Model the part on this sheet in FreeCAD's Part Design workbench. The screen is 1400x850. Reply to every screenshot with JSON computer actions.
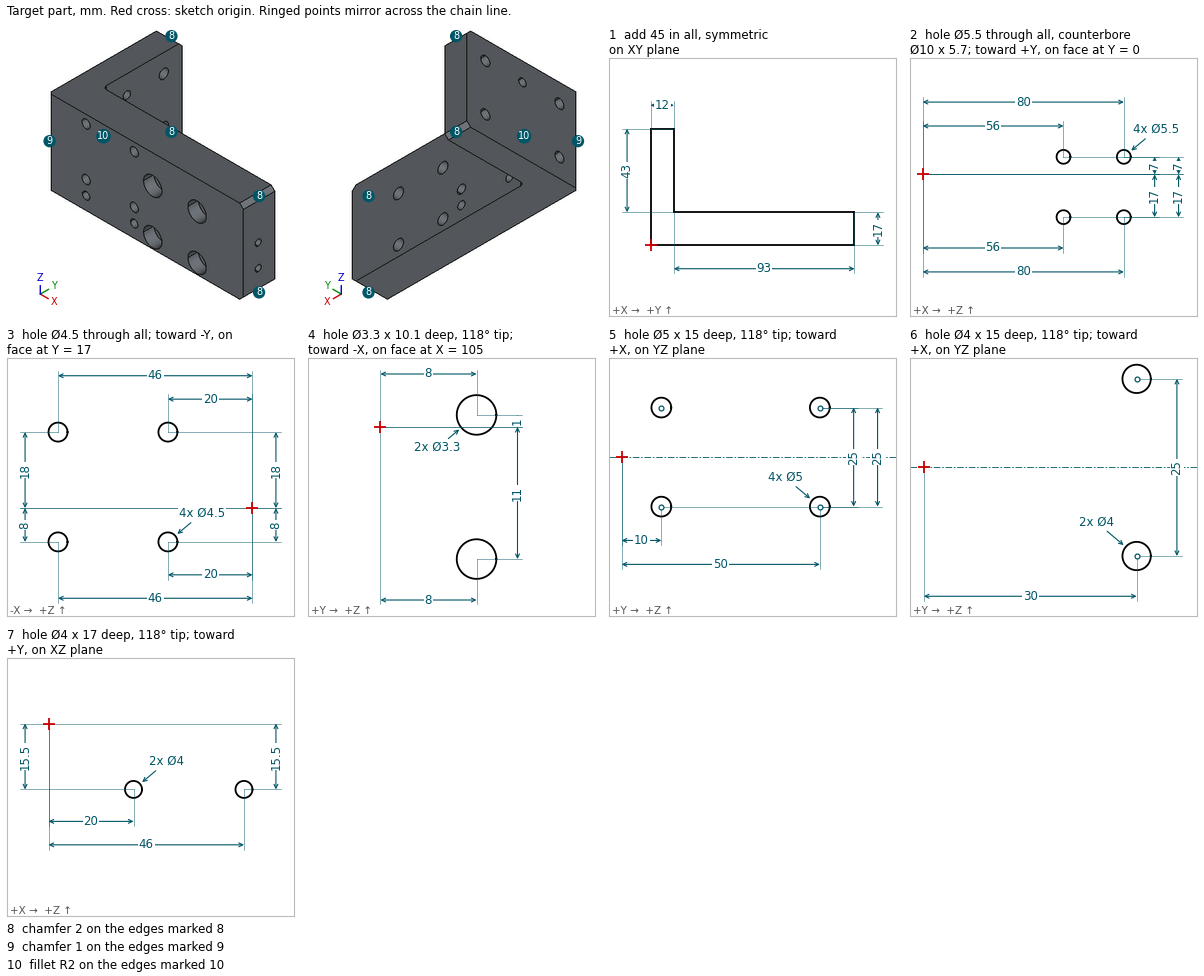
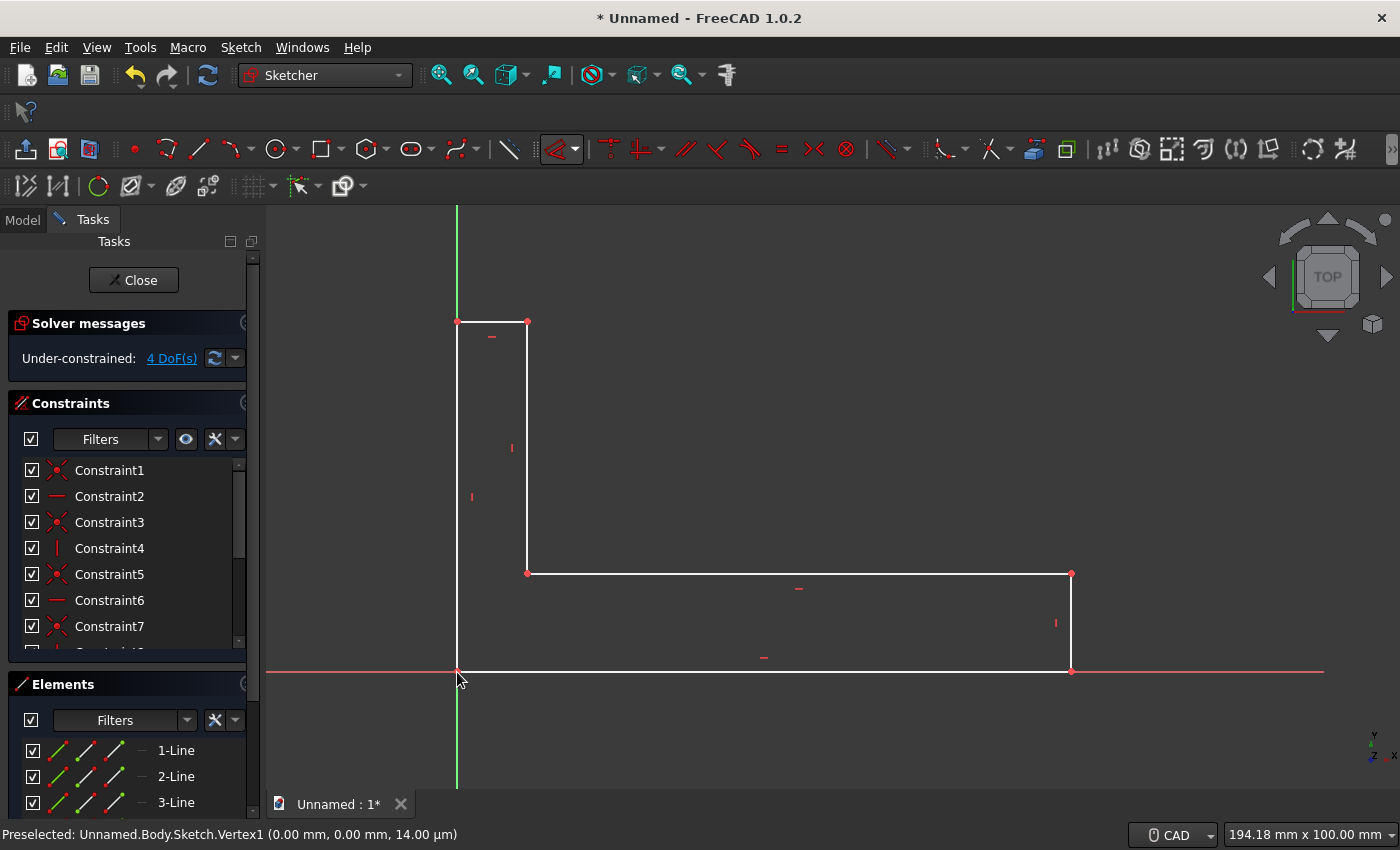
{"action": "left_click", "coordinate": [1071, 643]}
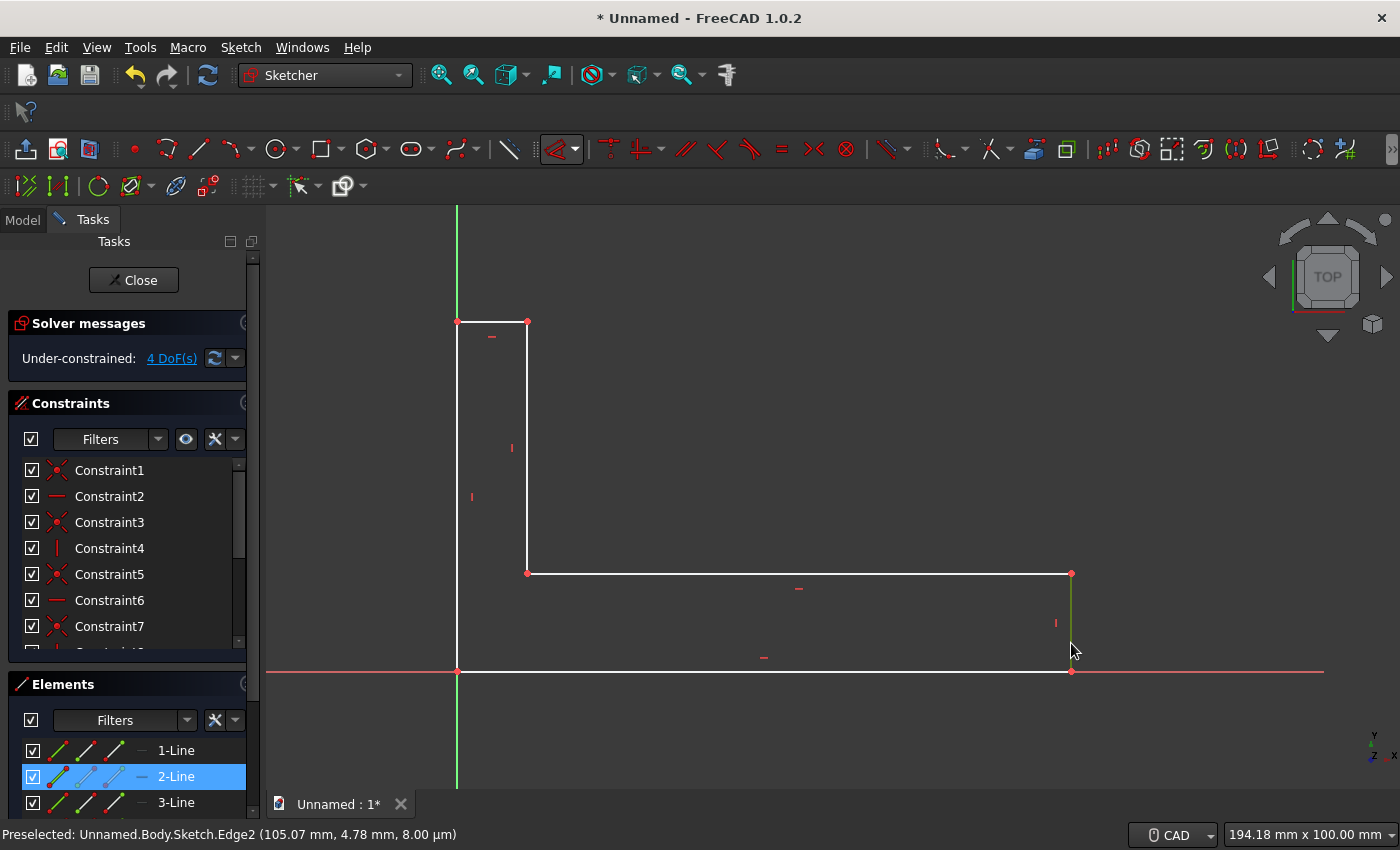
{"action": "key", "text": "i"}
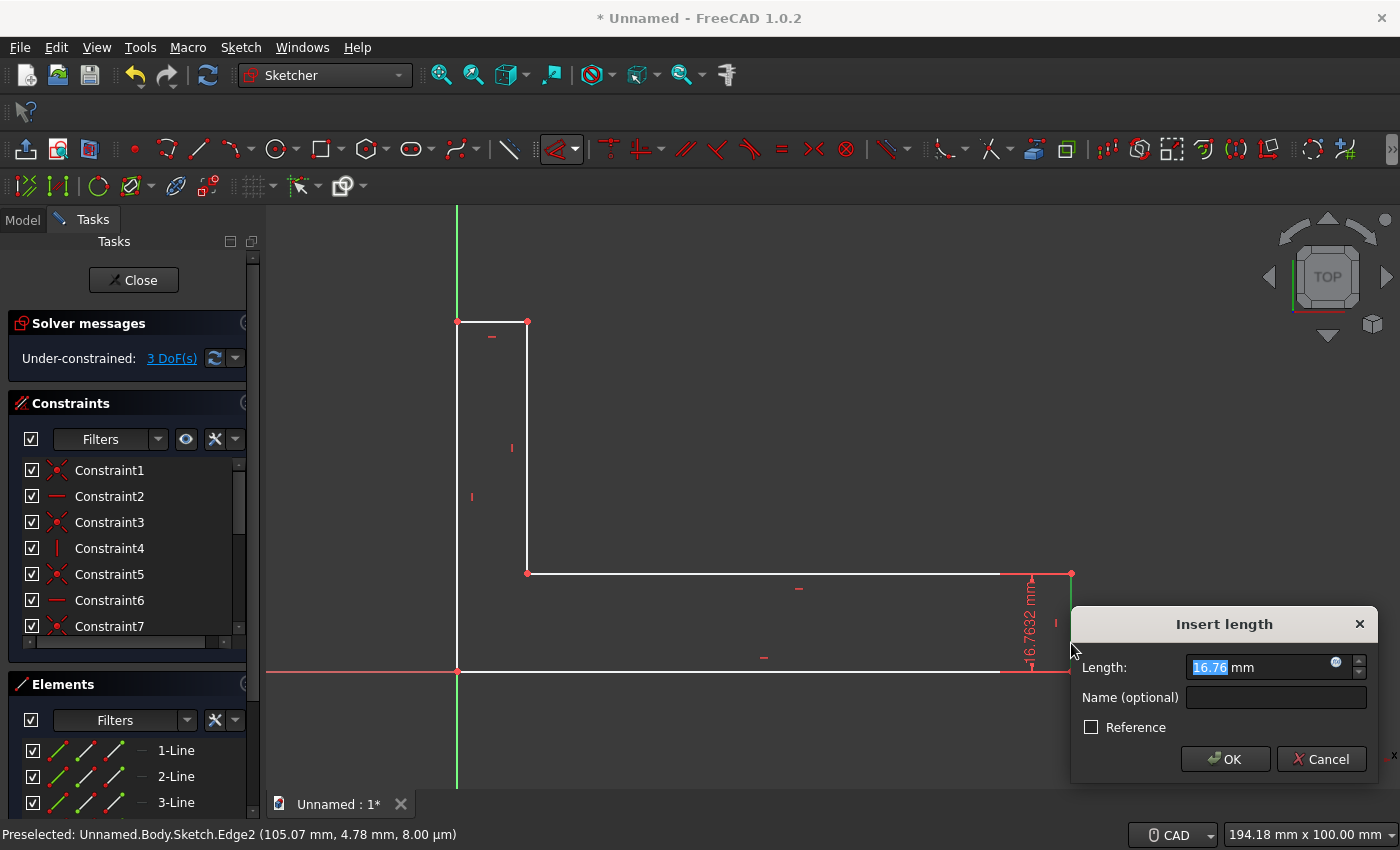
{"action": "type", "text": "17"}
{"action": "key", "text": "Return"}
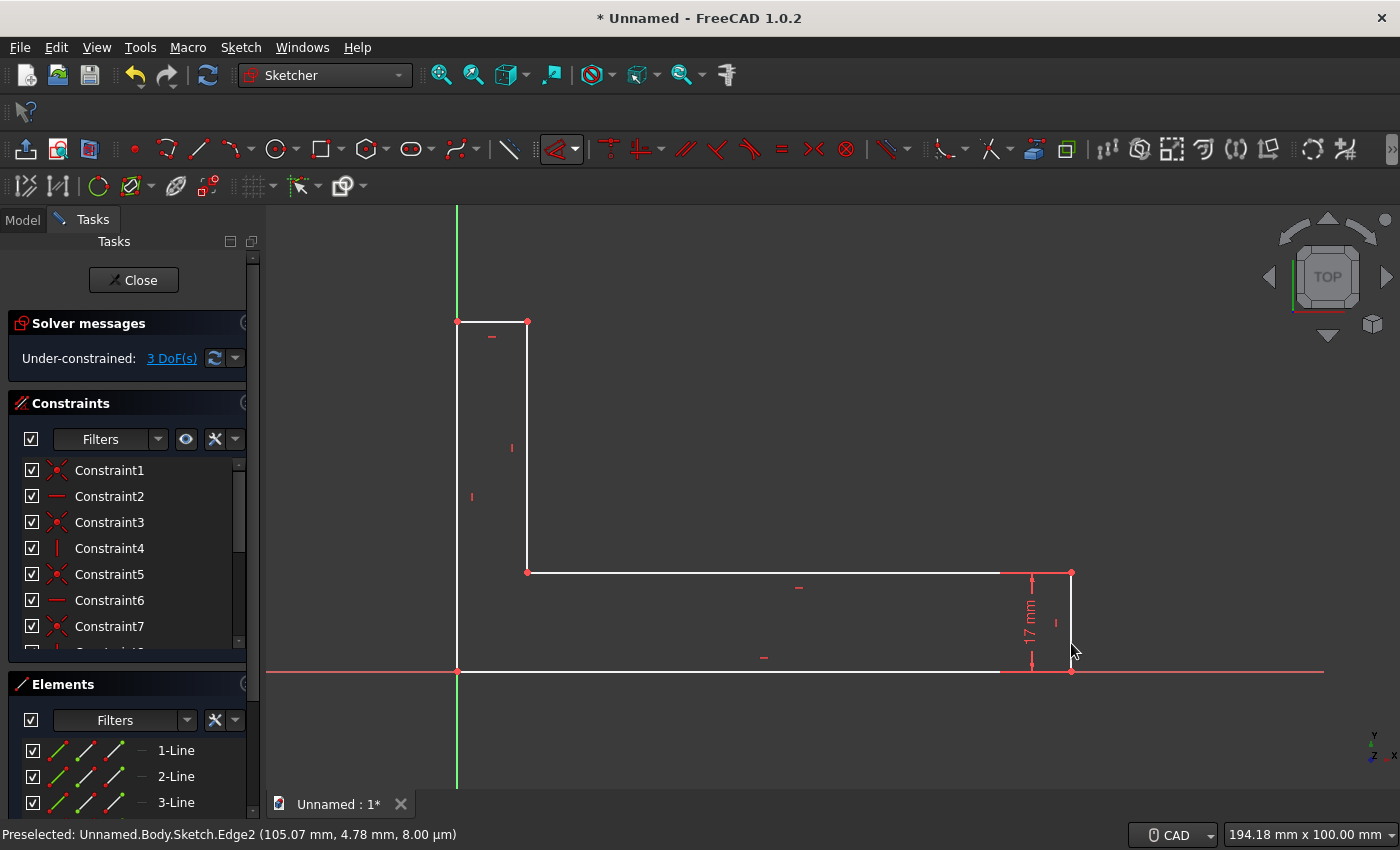
{"action": "left_click", "coordinate": [908, 573]}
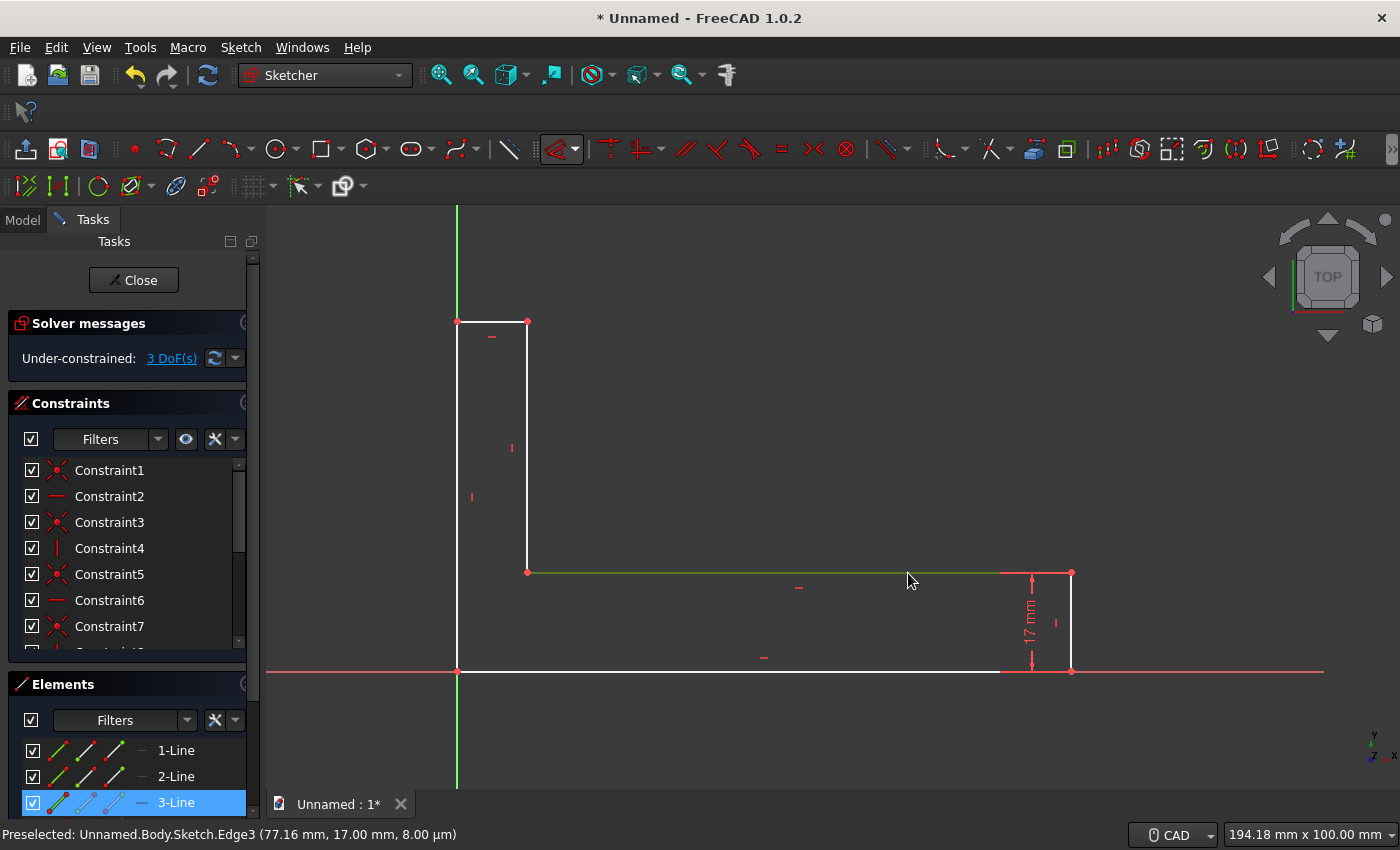
{"action": "key", "text": "l"}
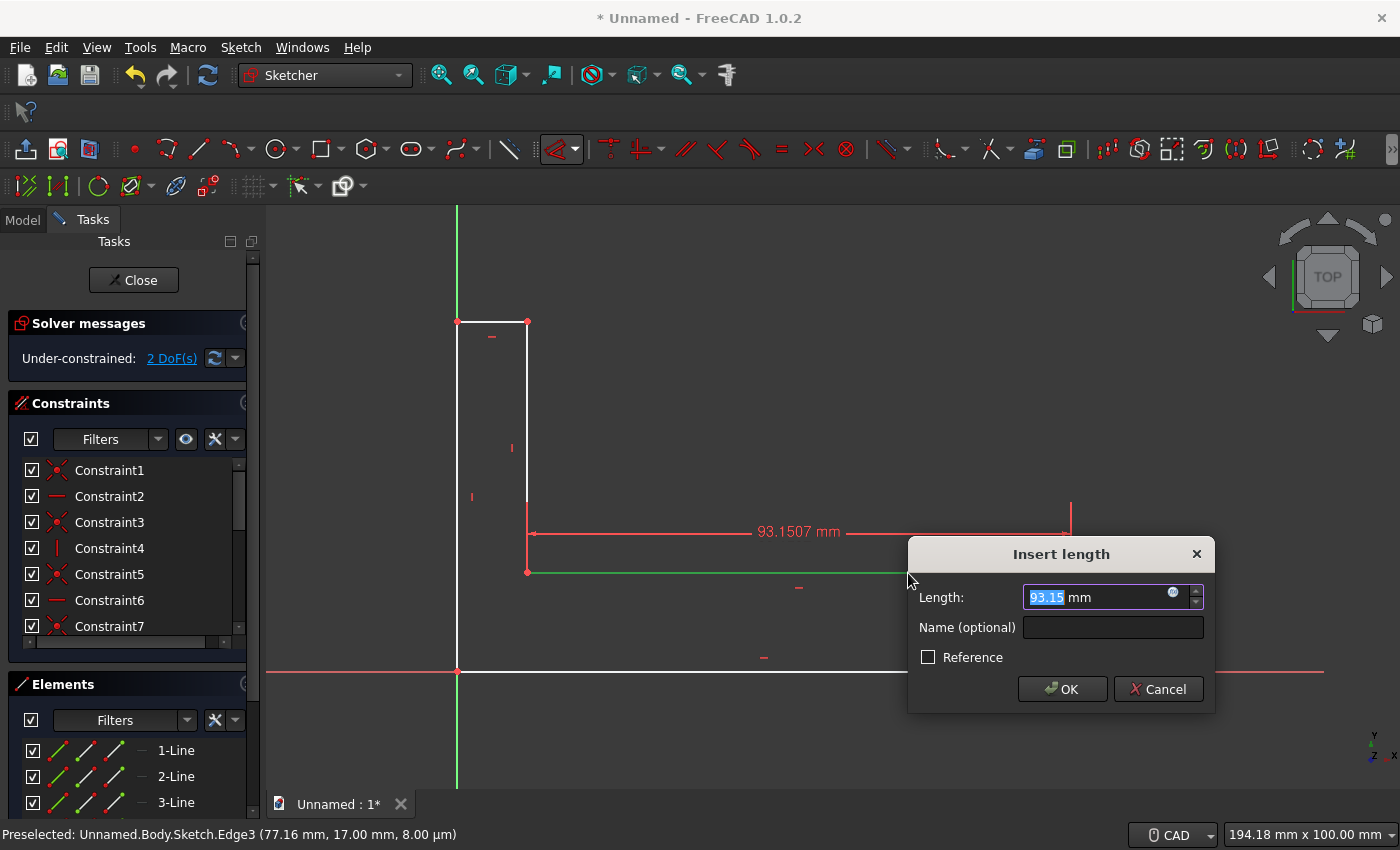
{"action": "type", "text": "93"}
{"action": "key", "text": "Return"}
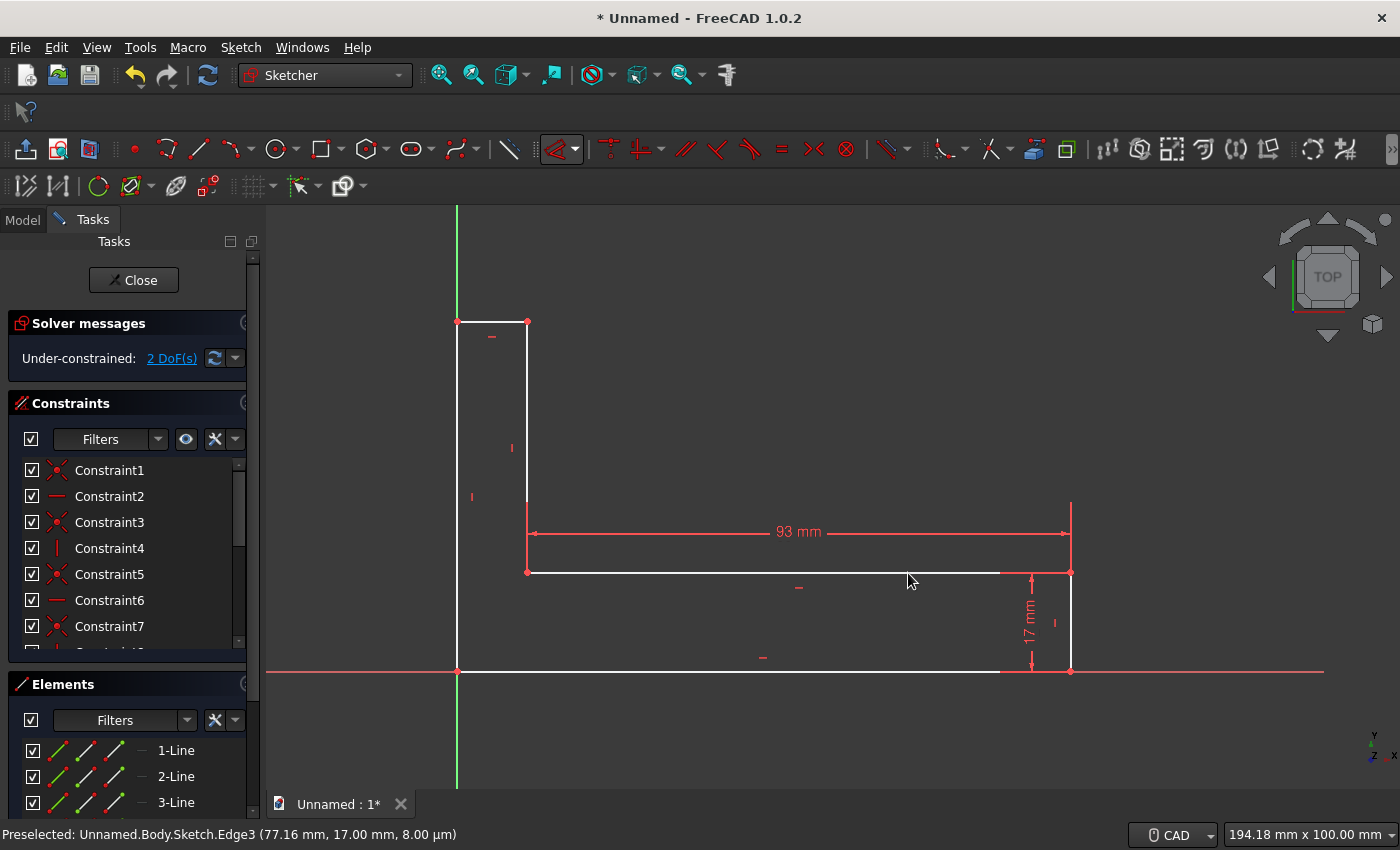
{"action": "left_click", "coordinate": [527, 497]}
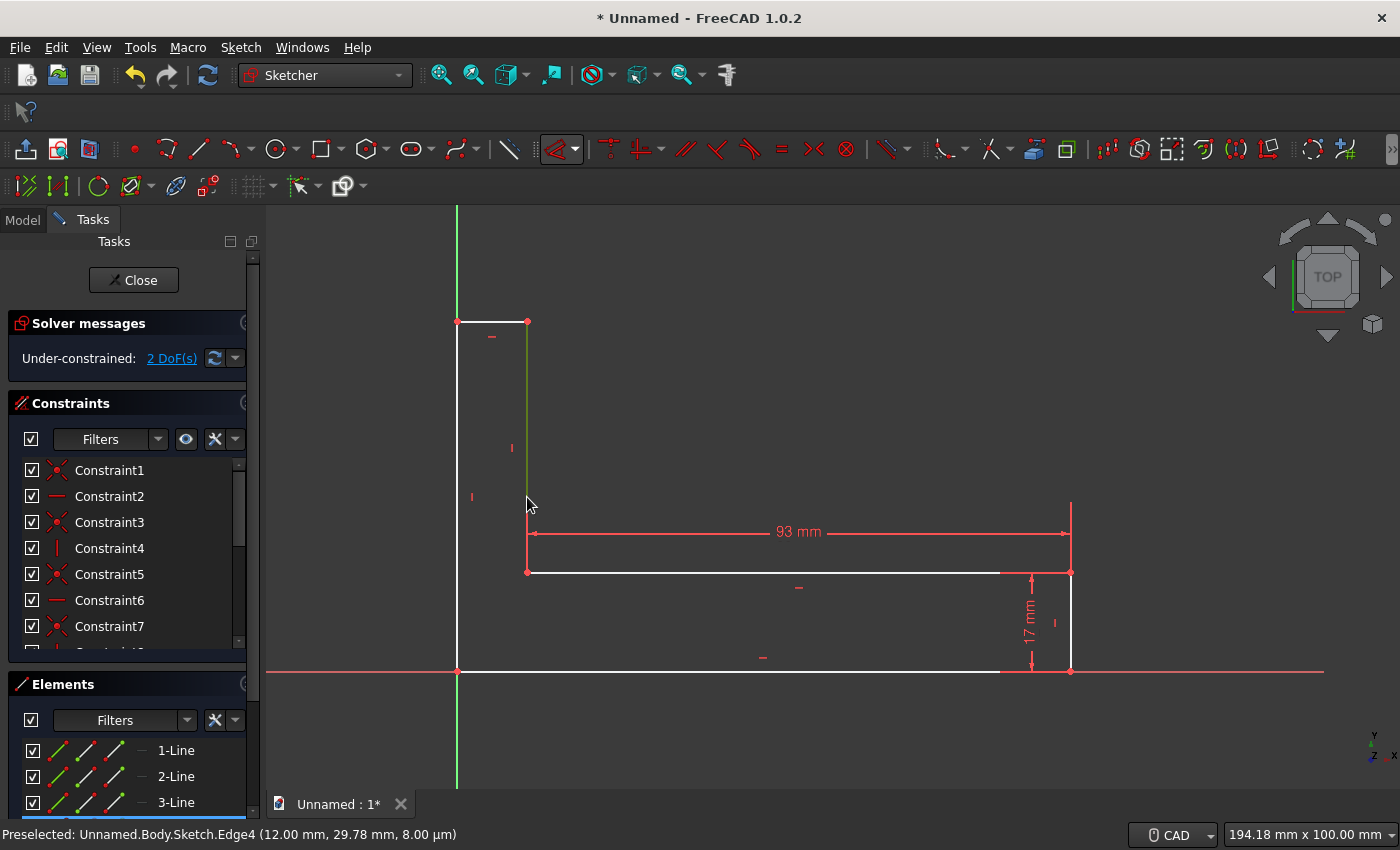
{"action": "key", "text": "i"}